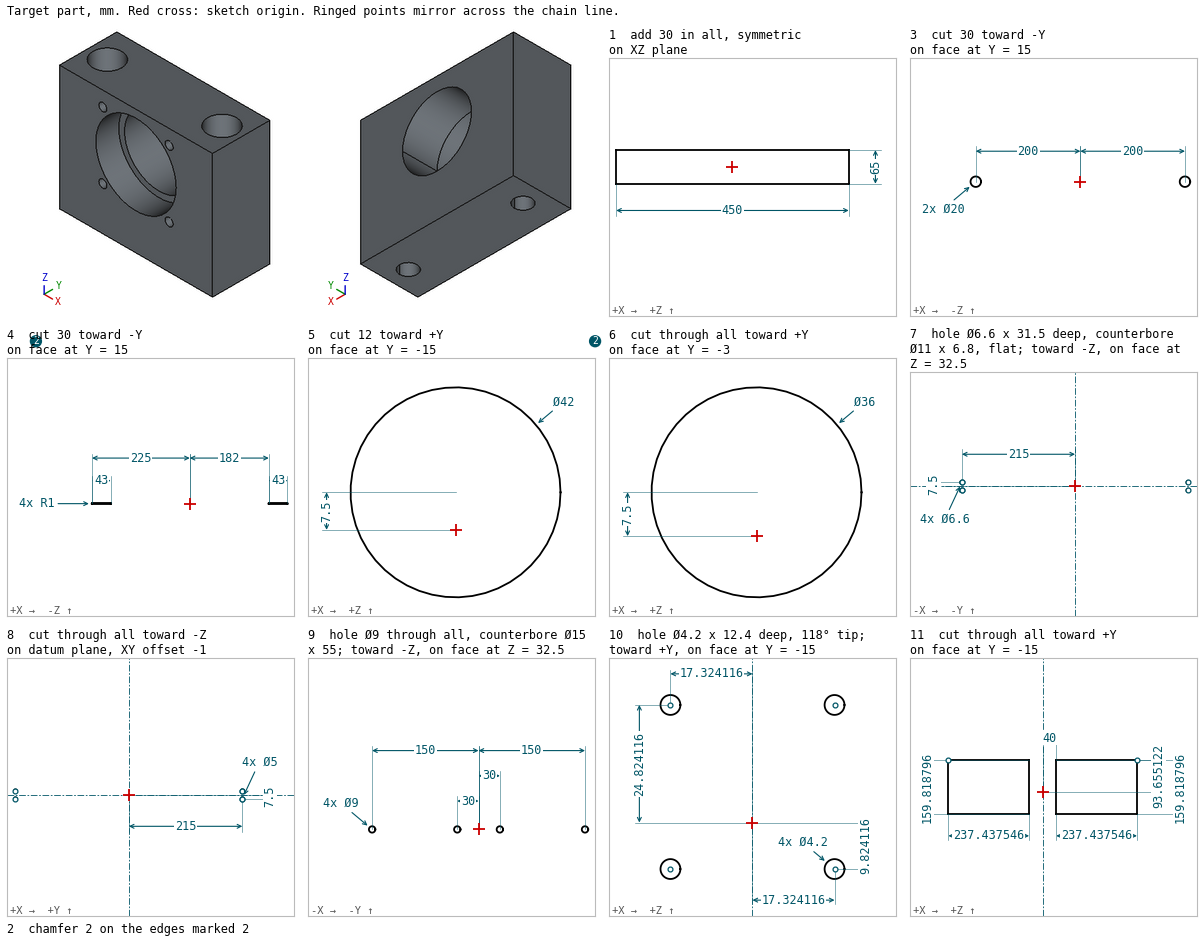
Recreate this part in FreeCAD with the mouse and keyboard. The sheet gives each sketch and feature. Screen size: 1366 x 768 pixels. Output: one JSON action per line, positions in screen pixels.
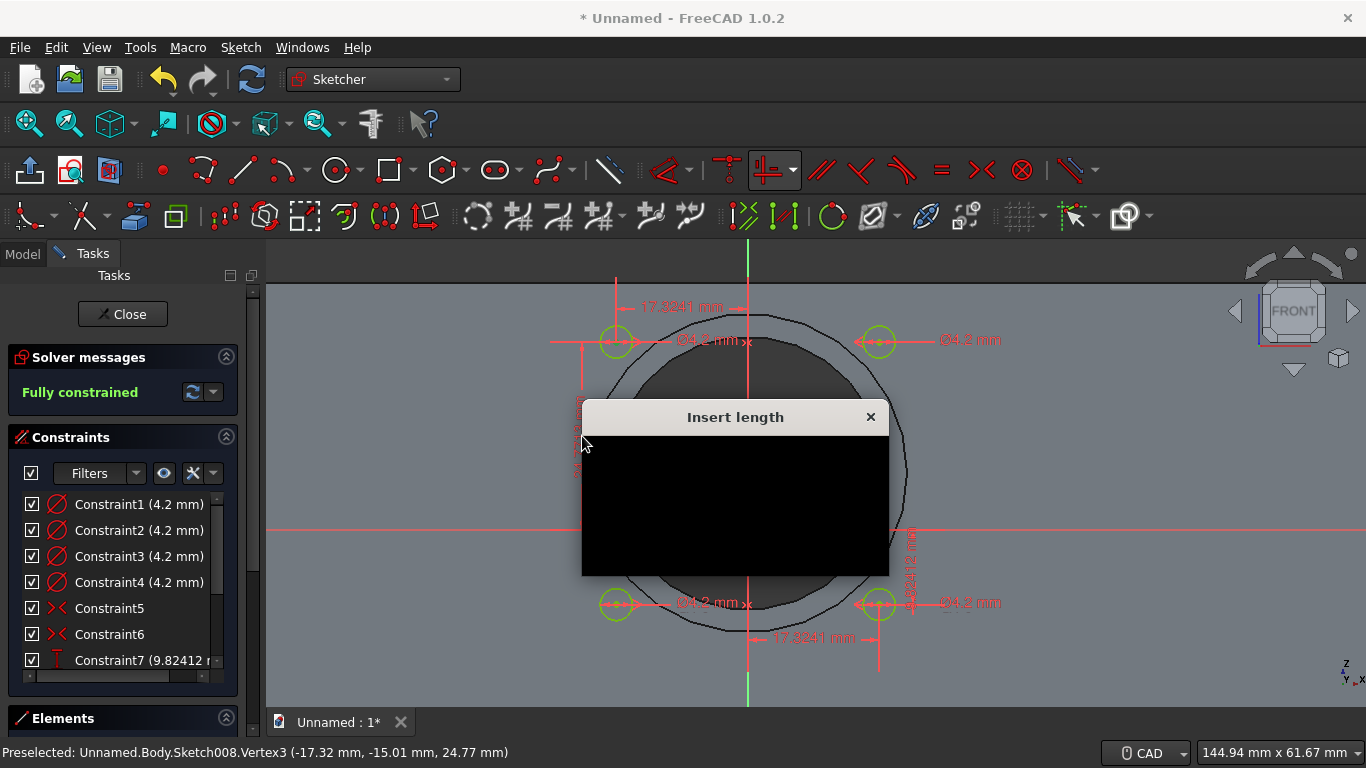
{"action": "type", "text": "24.824116"}
{"action": "key", "text": "Return"}
{"action": "key", "text": "Escape"}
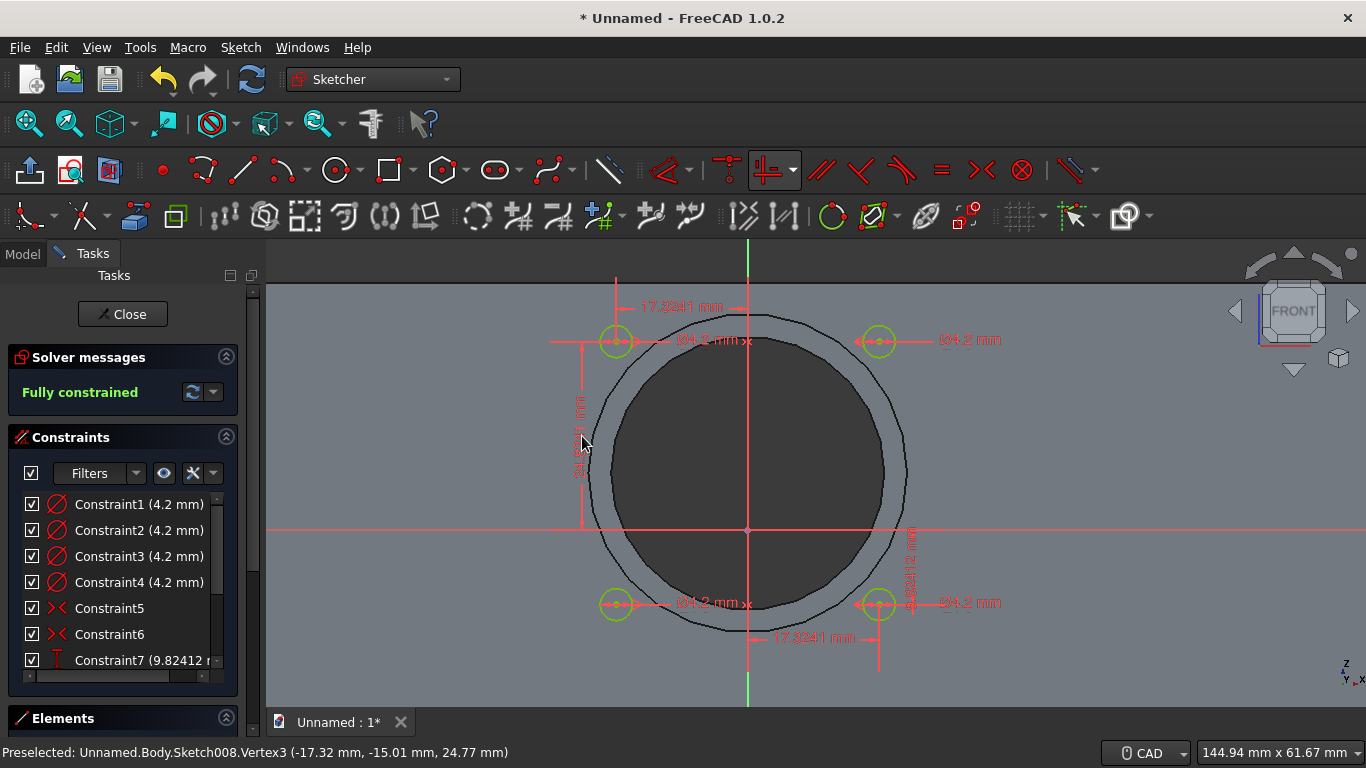
{"action": "left_click", "coordinate": [123, 314]}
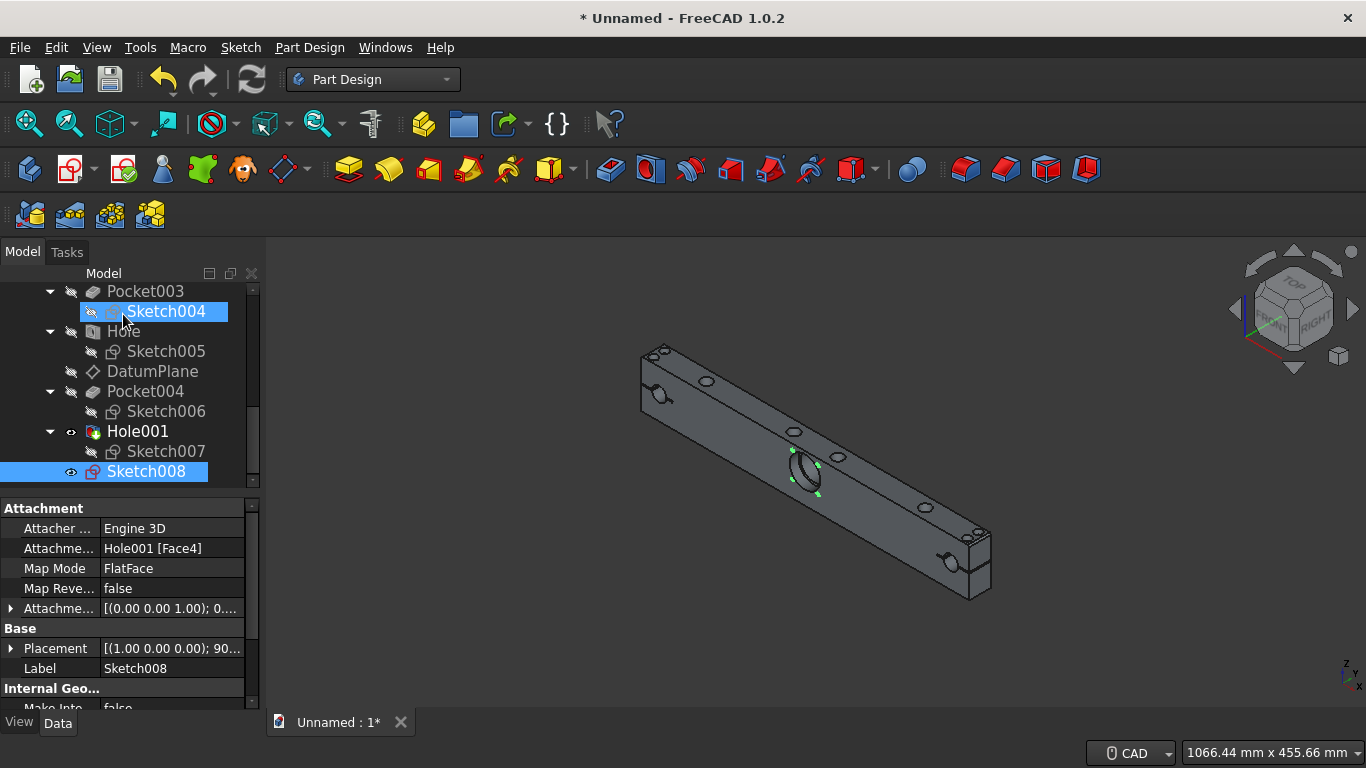
{"action": "left_click", "coordinate": [652, 170]}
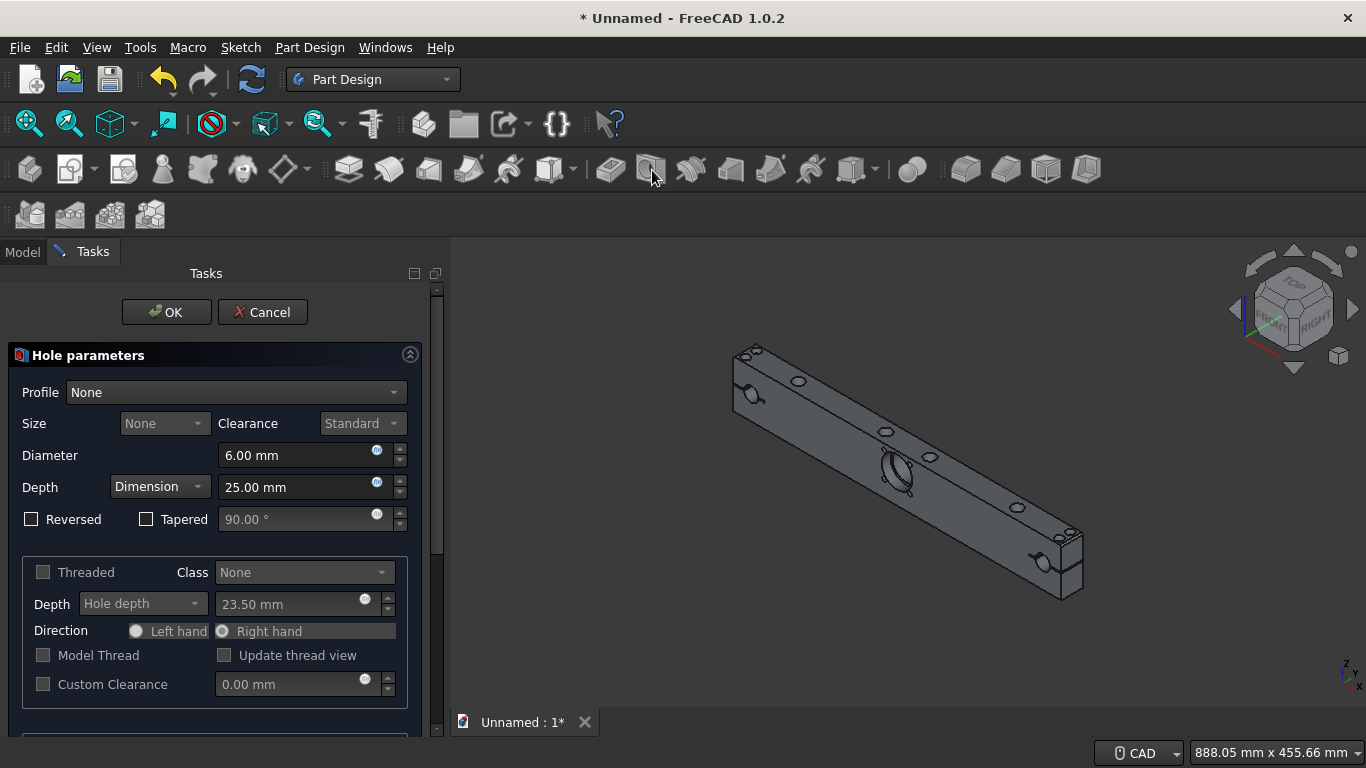
{"action": "triple_click", "coordinate": [305, 455]}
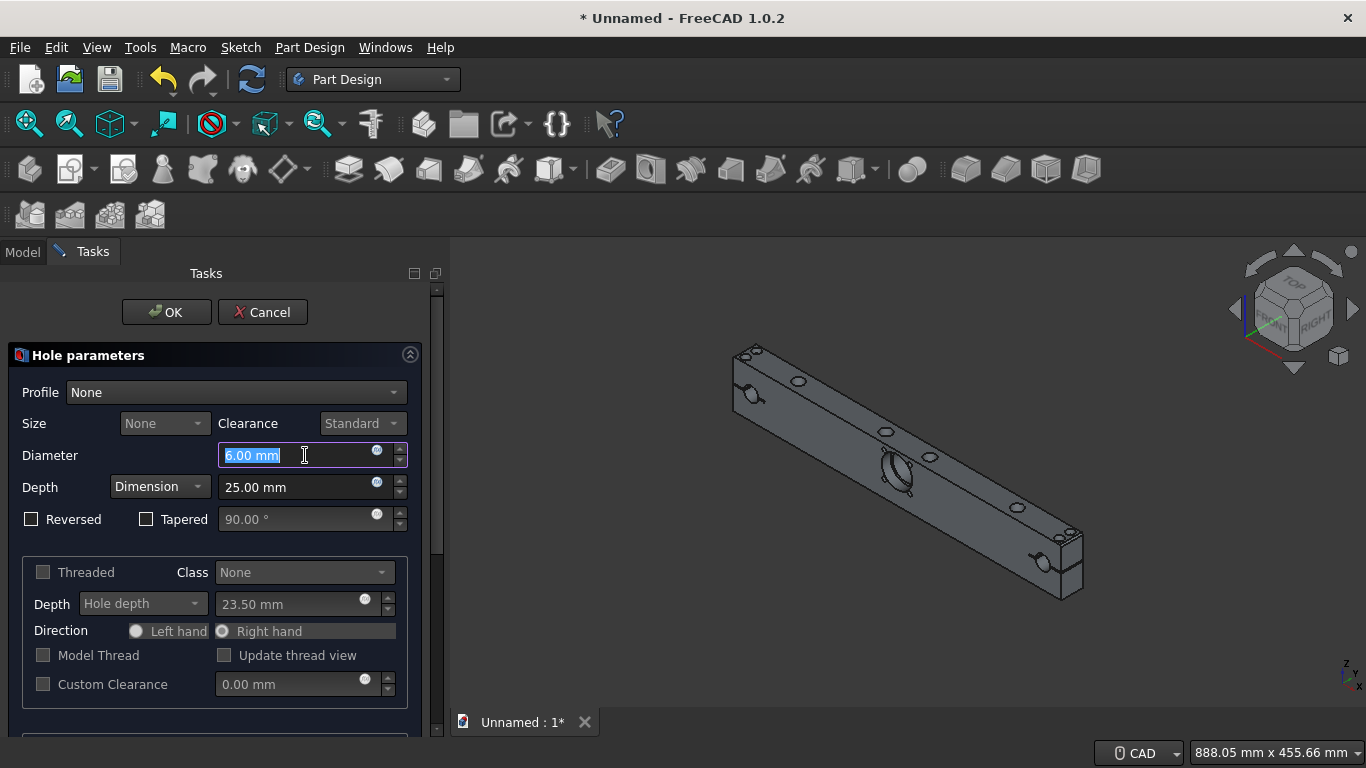
{"action": "type", "text": "4.2"}
{"action": "key", "text": "Tab"}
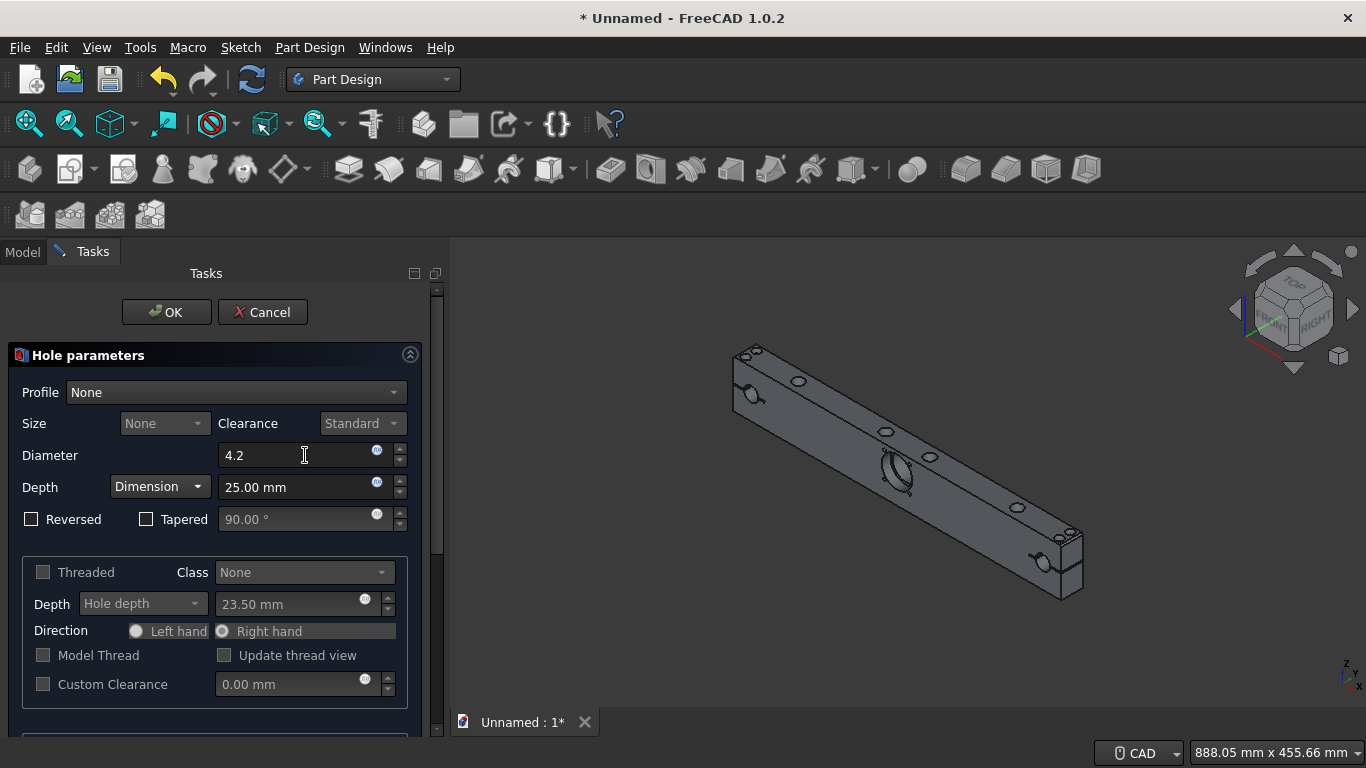
{"action": "triple_click", "coordinate": [305, 487]}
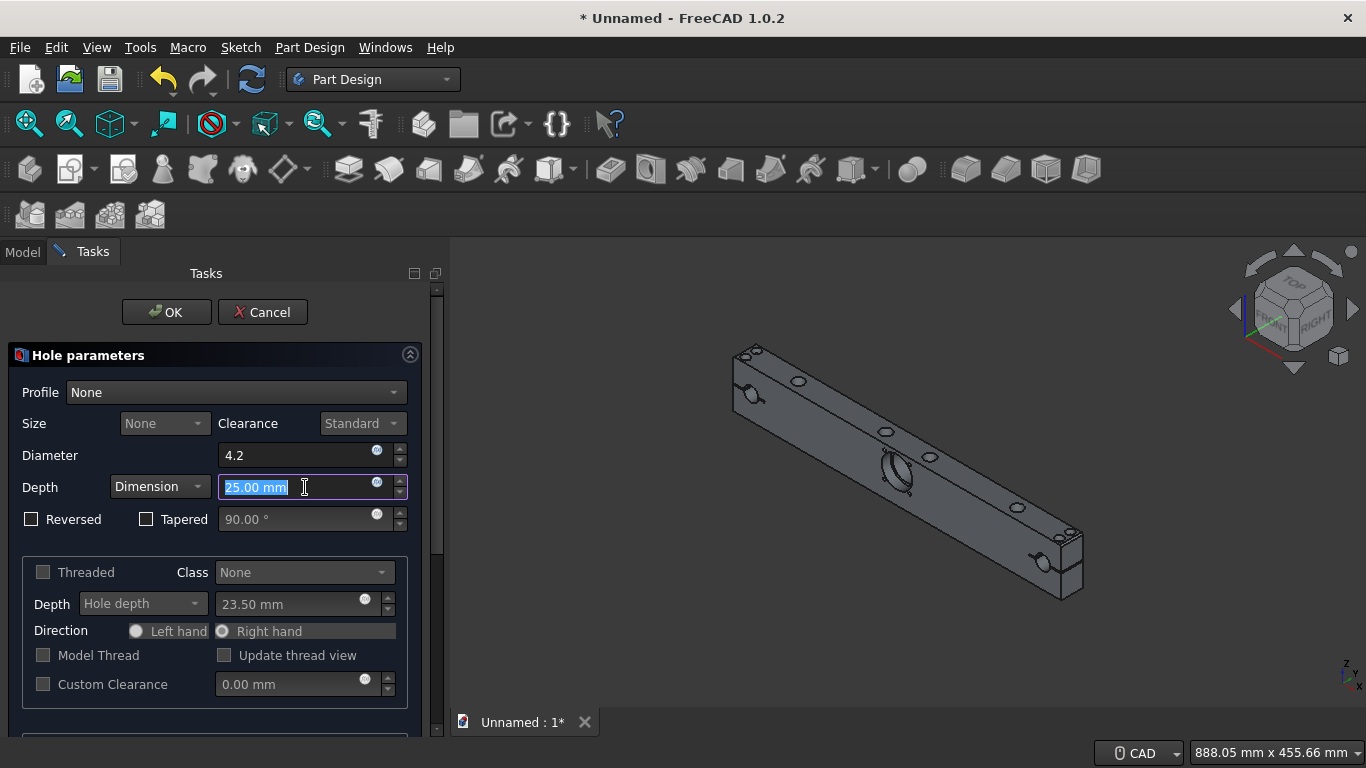
{"action": "type", "text": "12.4"}
{"action": "key", "text": "Tab"}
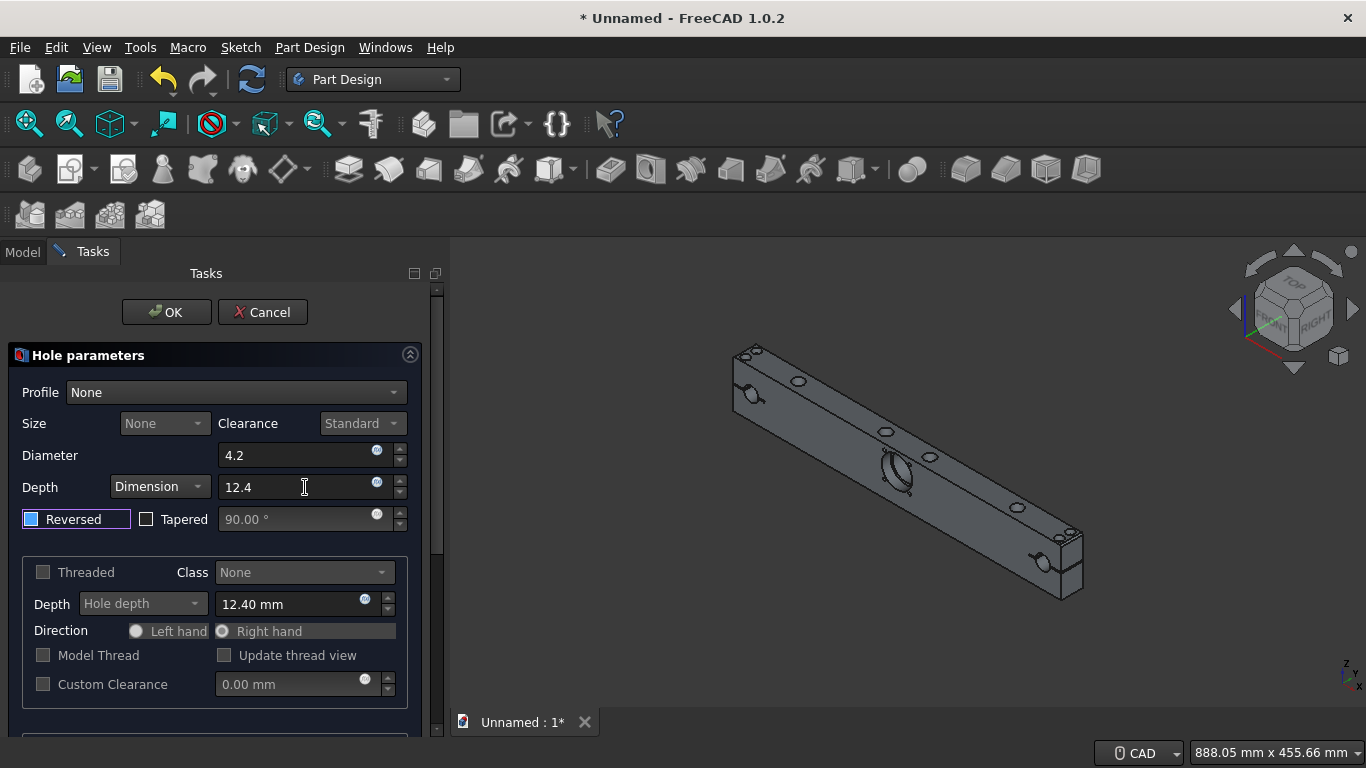
{"action": "left_click", "coordinate": [167, 312]}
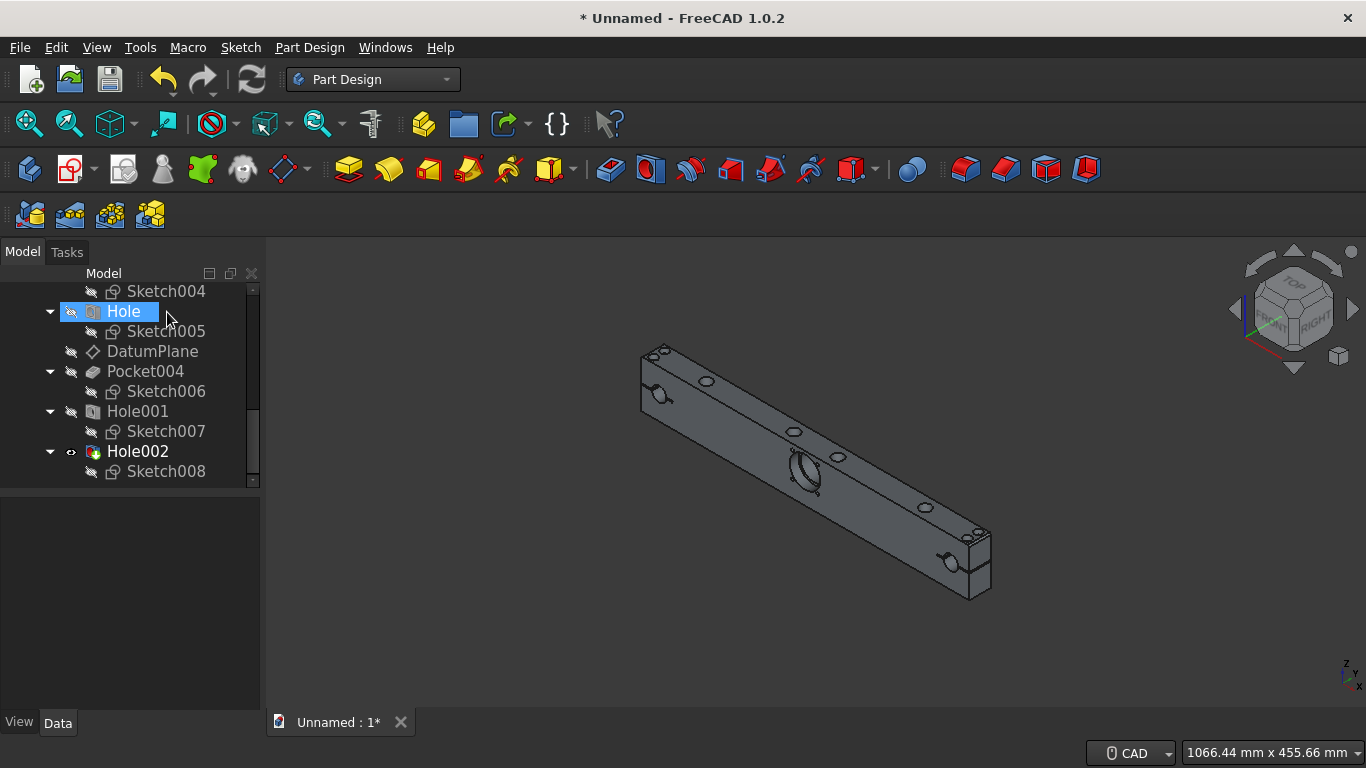
{"action": "left_click", "coordinate": [899, 531]}